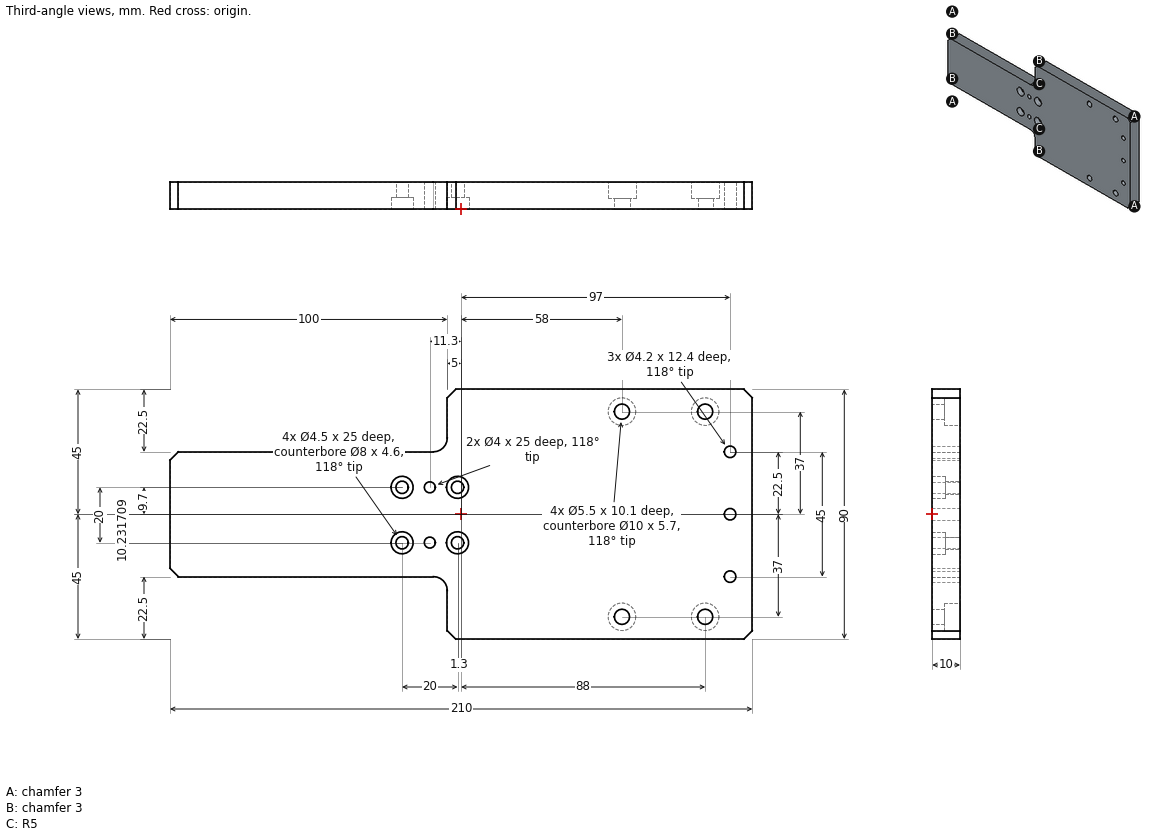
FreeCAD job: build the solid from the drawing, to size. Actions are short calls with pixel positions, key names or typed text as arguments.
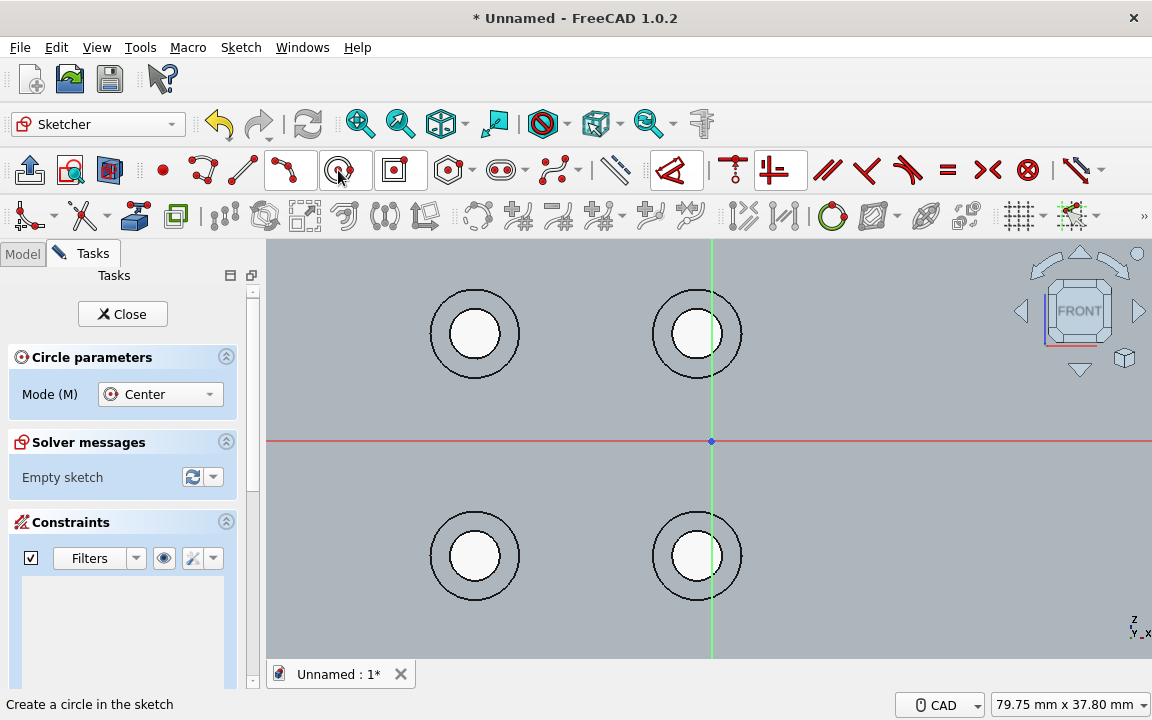
click(586, 334)
click(602, 318)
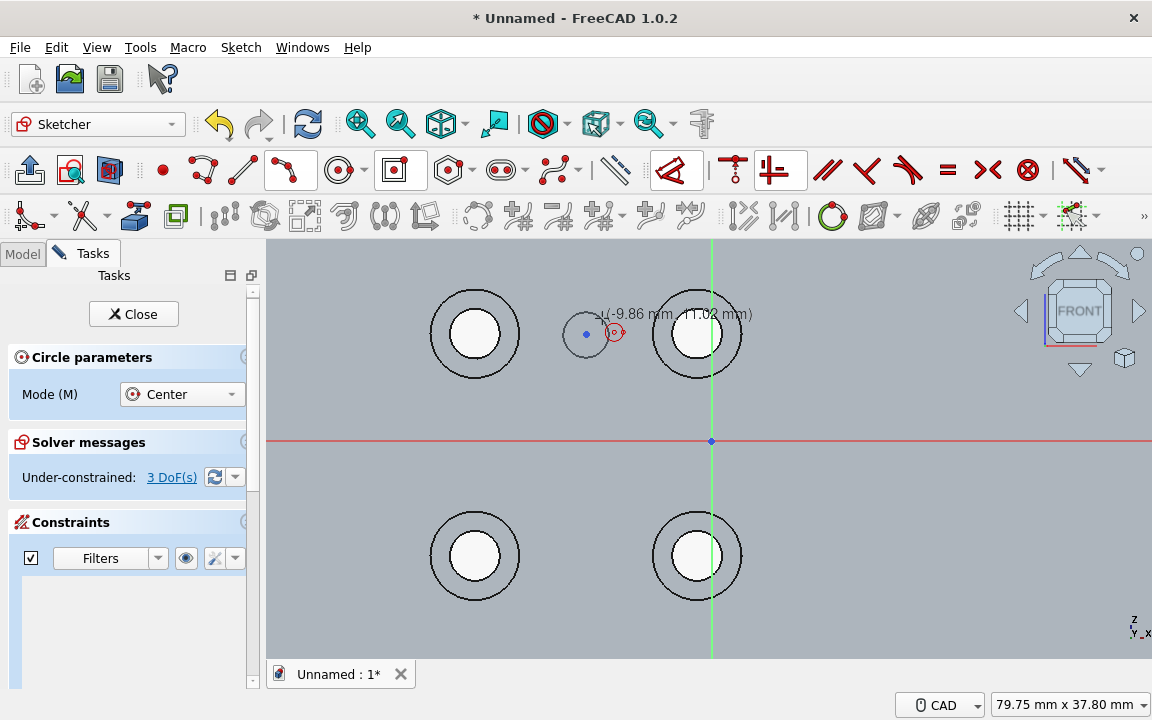
click(586, 555)
click(602, 539)
key(Escape)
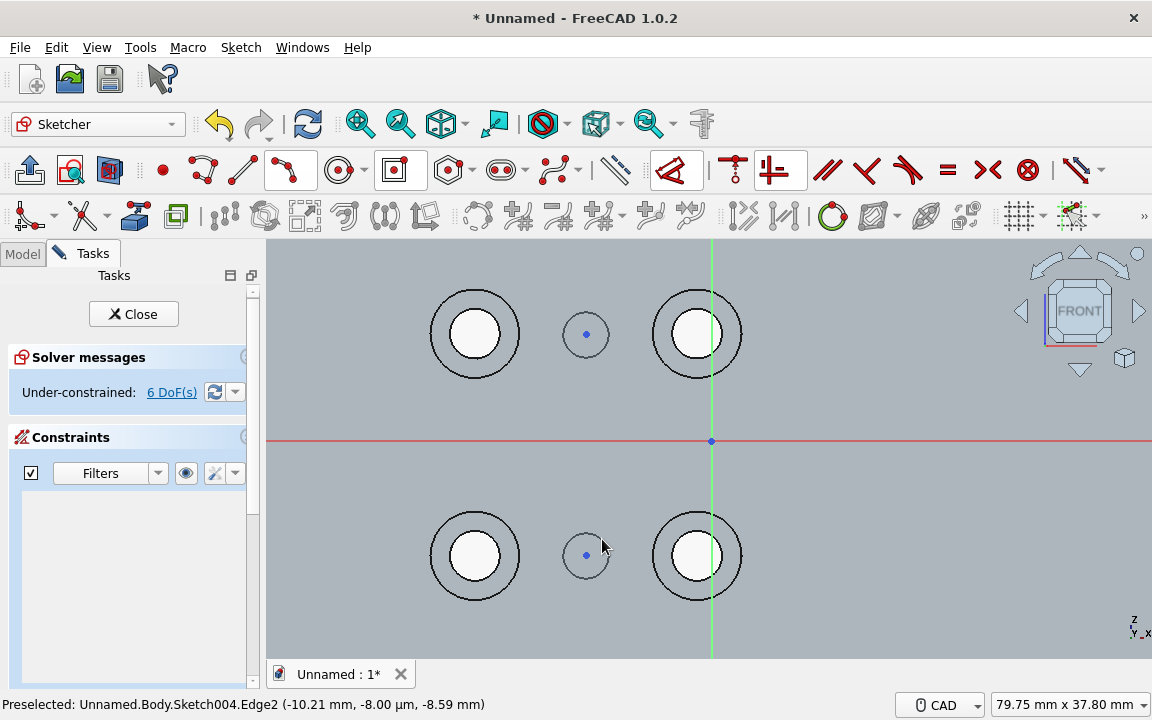
click(602, 319)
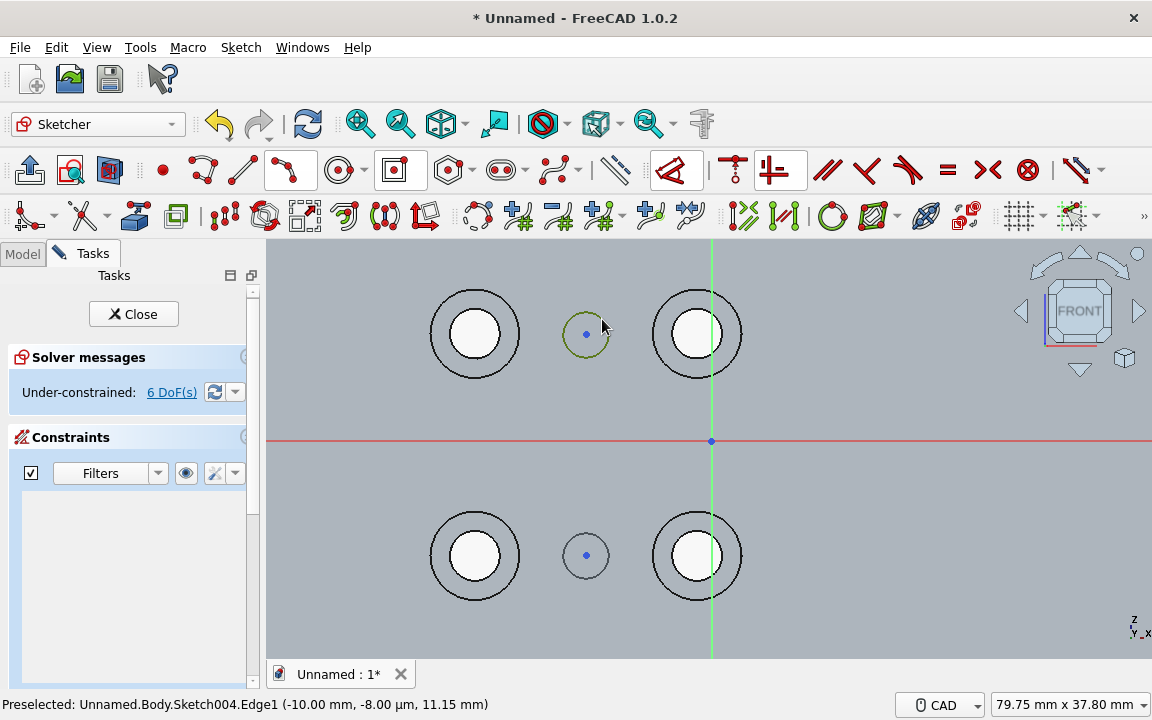
click(602, 540)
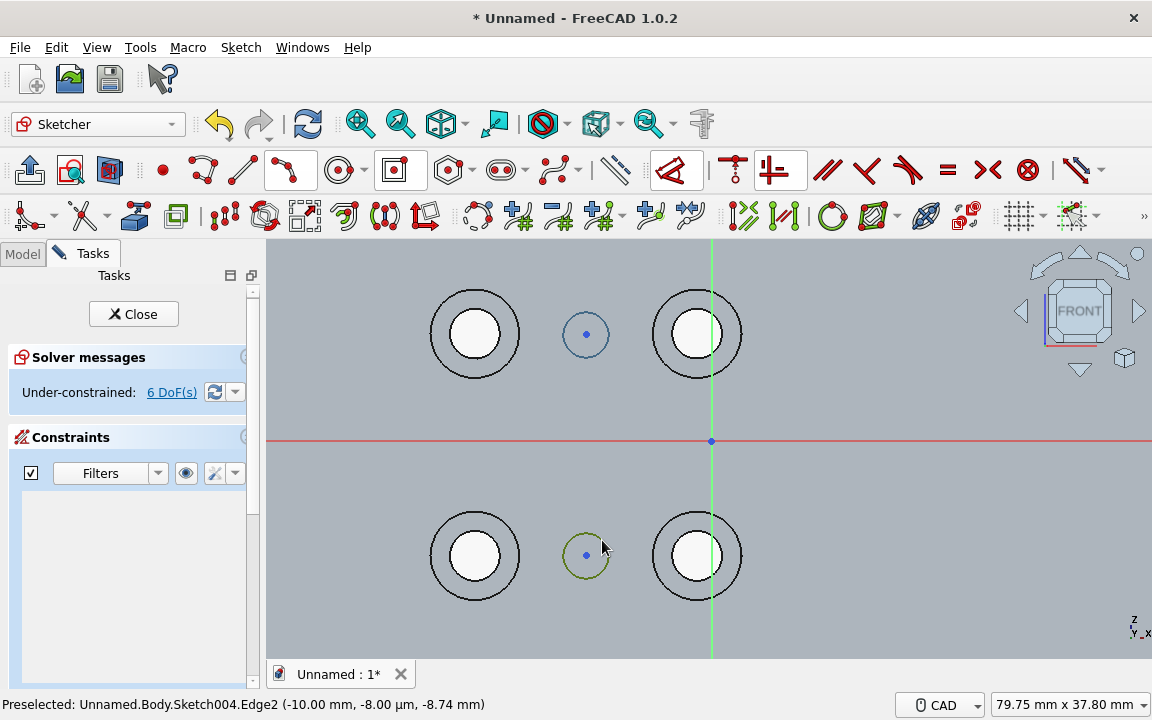
click(948, 170)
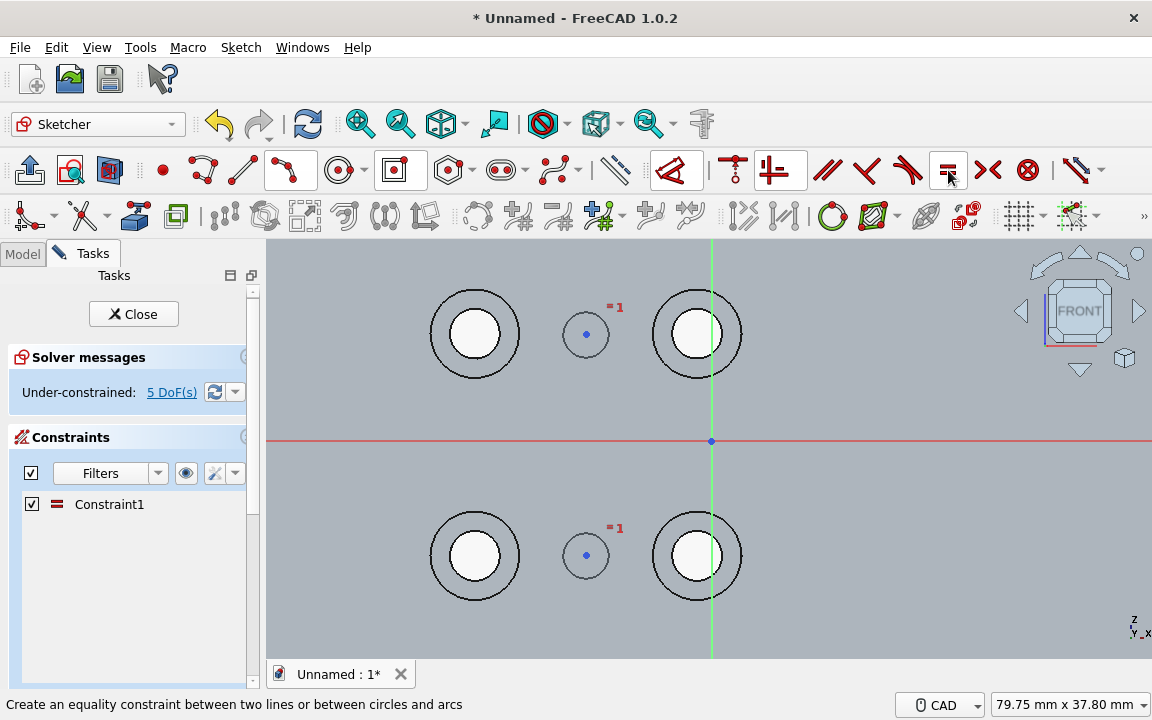
click(586, 335)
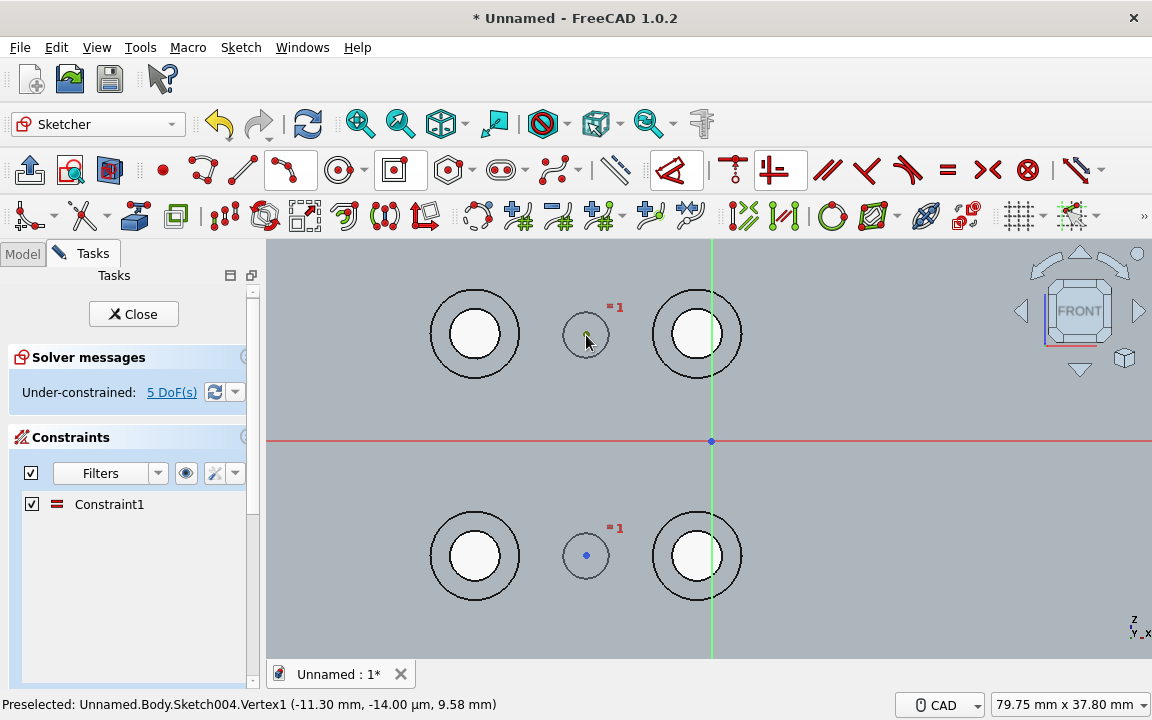
click(586, 556)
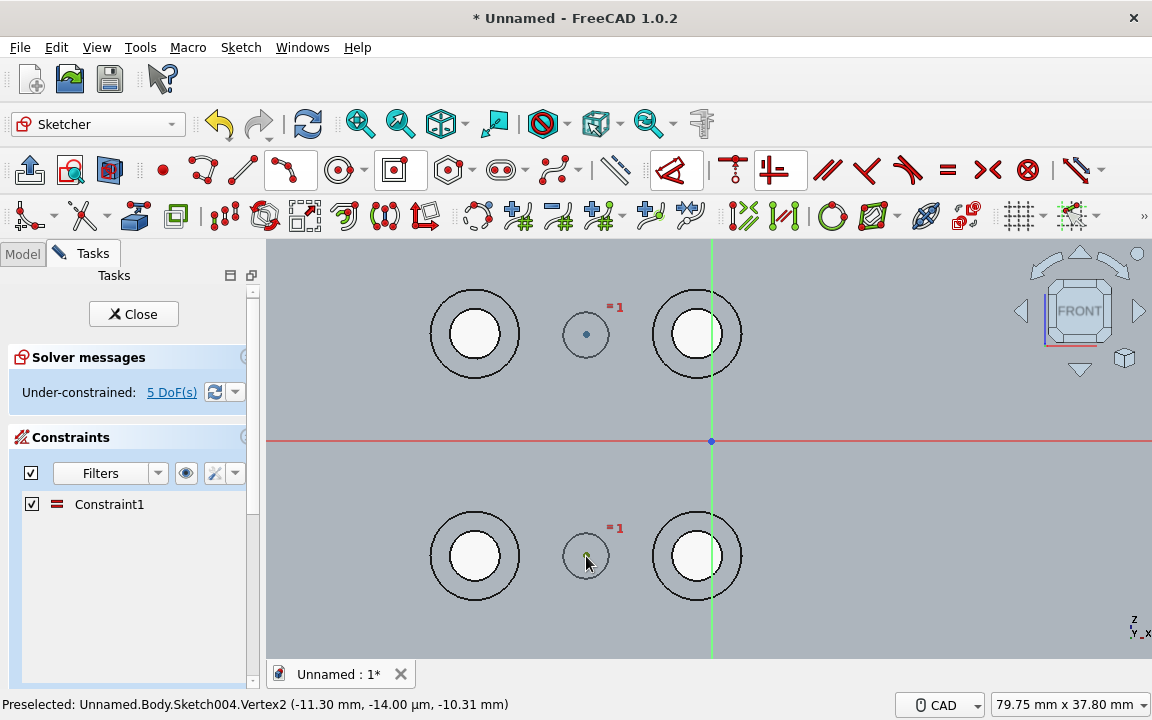
click(802, 170)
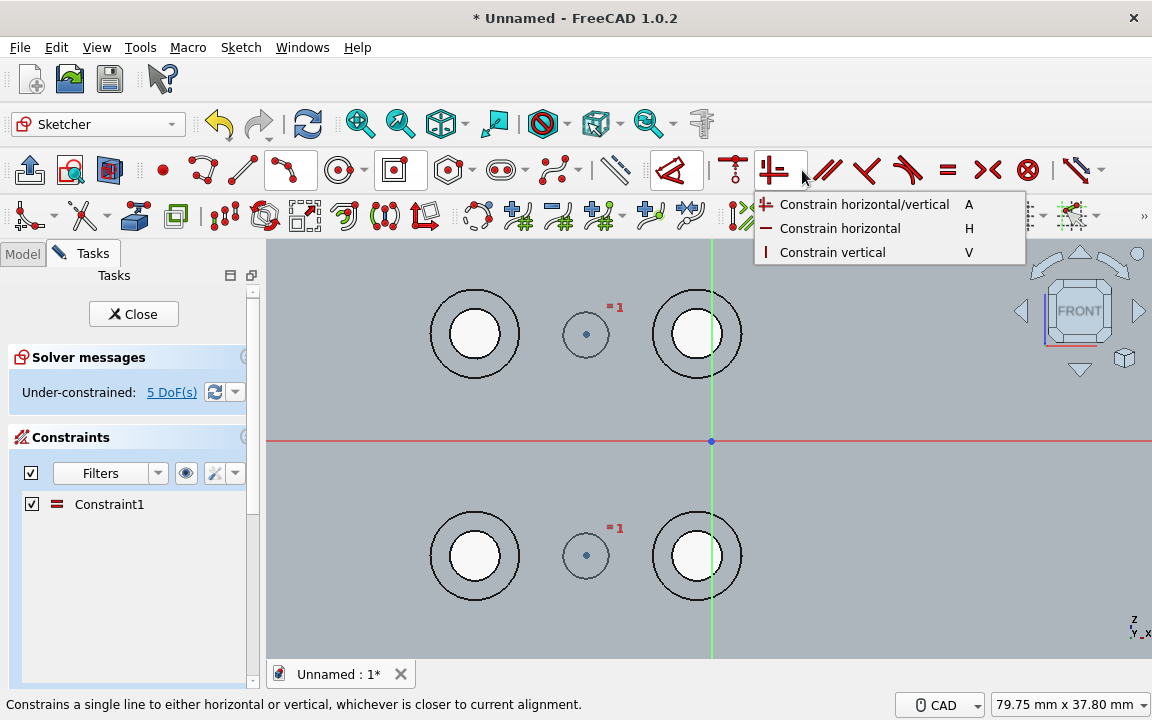
click(890, 252)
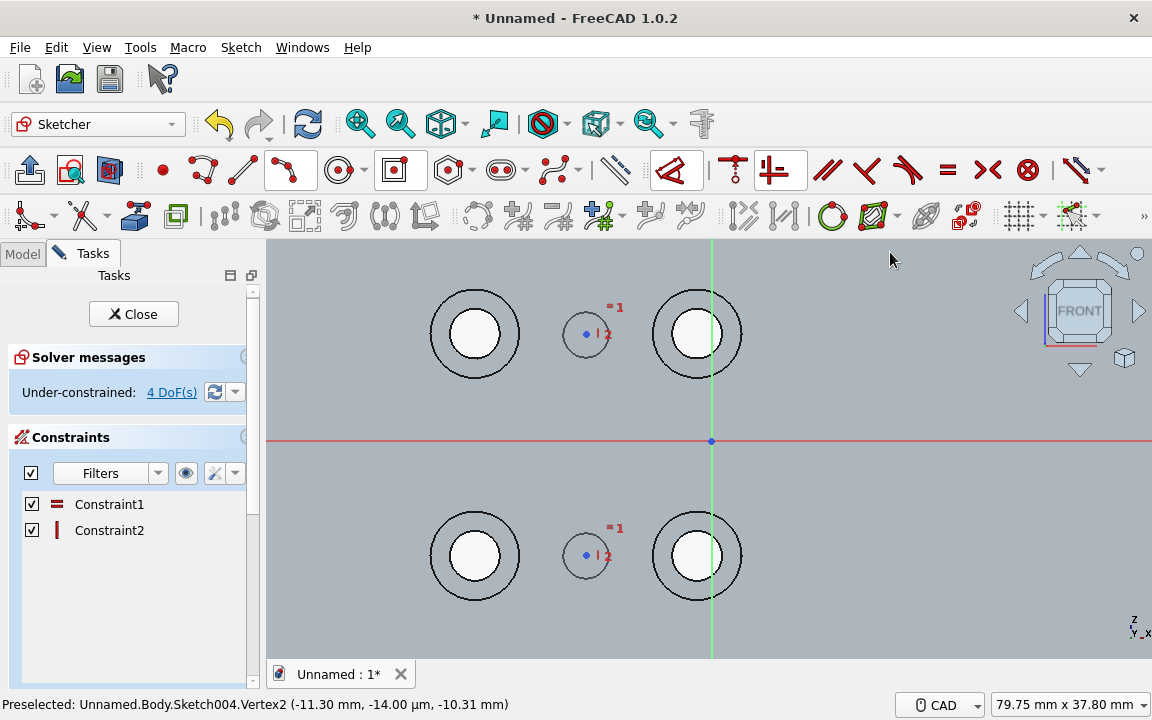
click(602, 319)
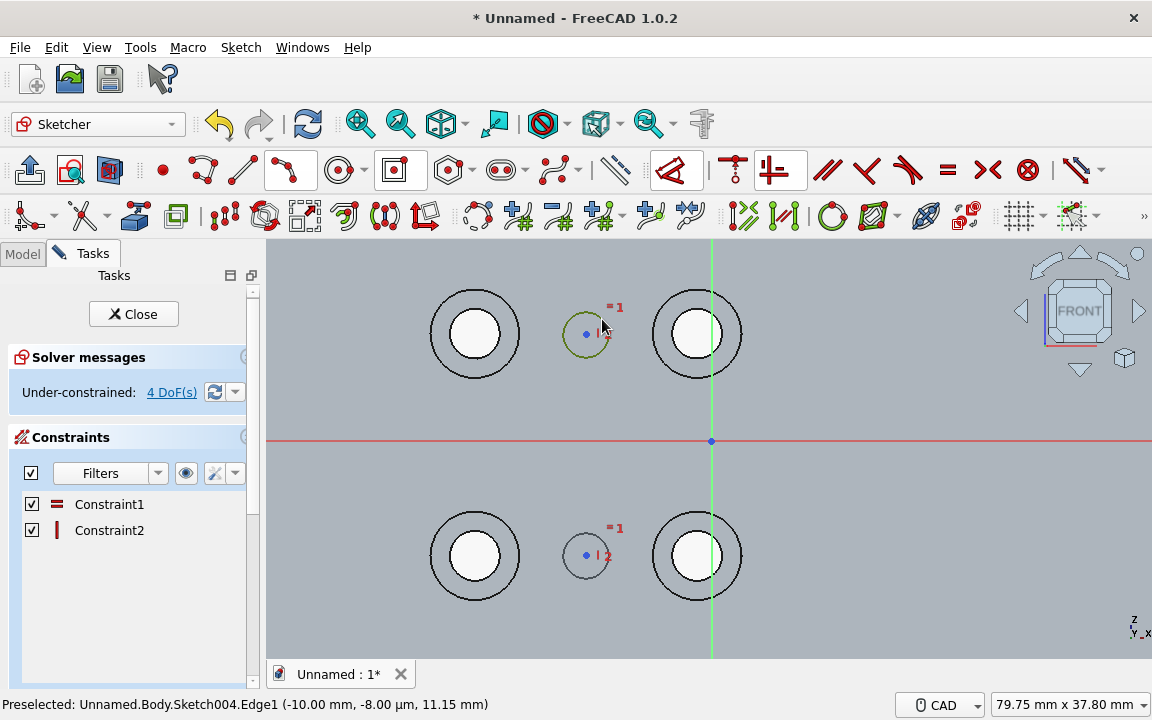
click(698, 170)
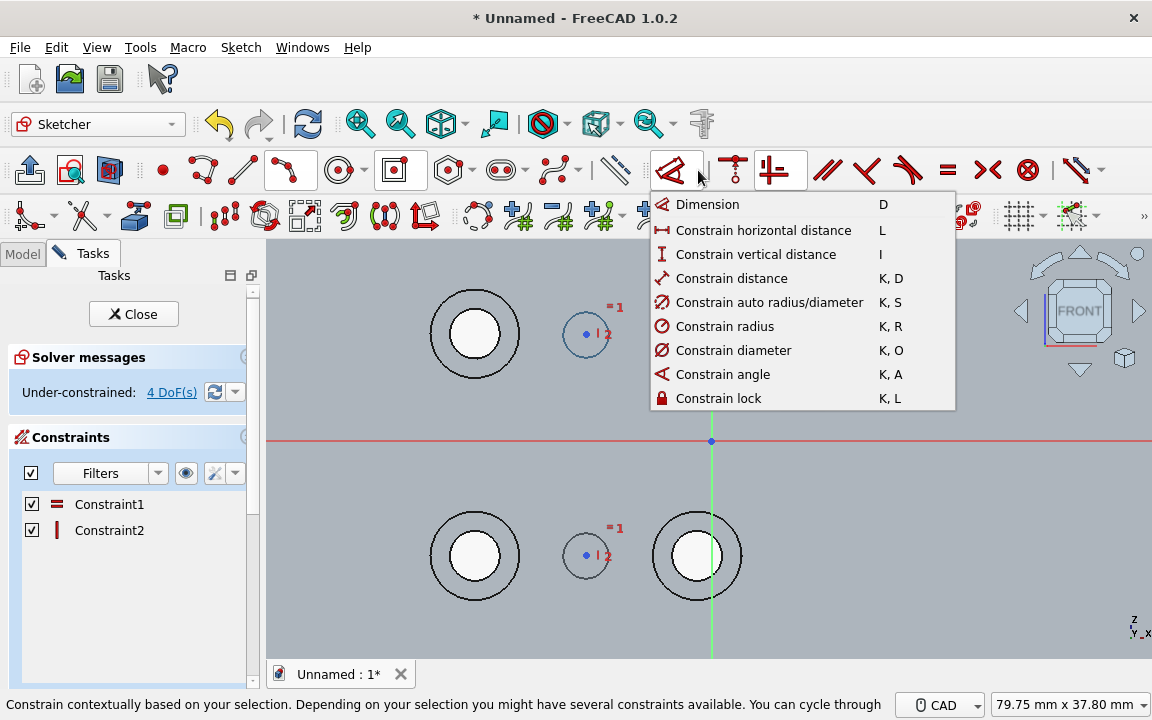
click(803, 350)